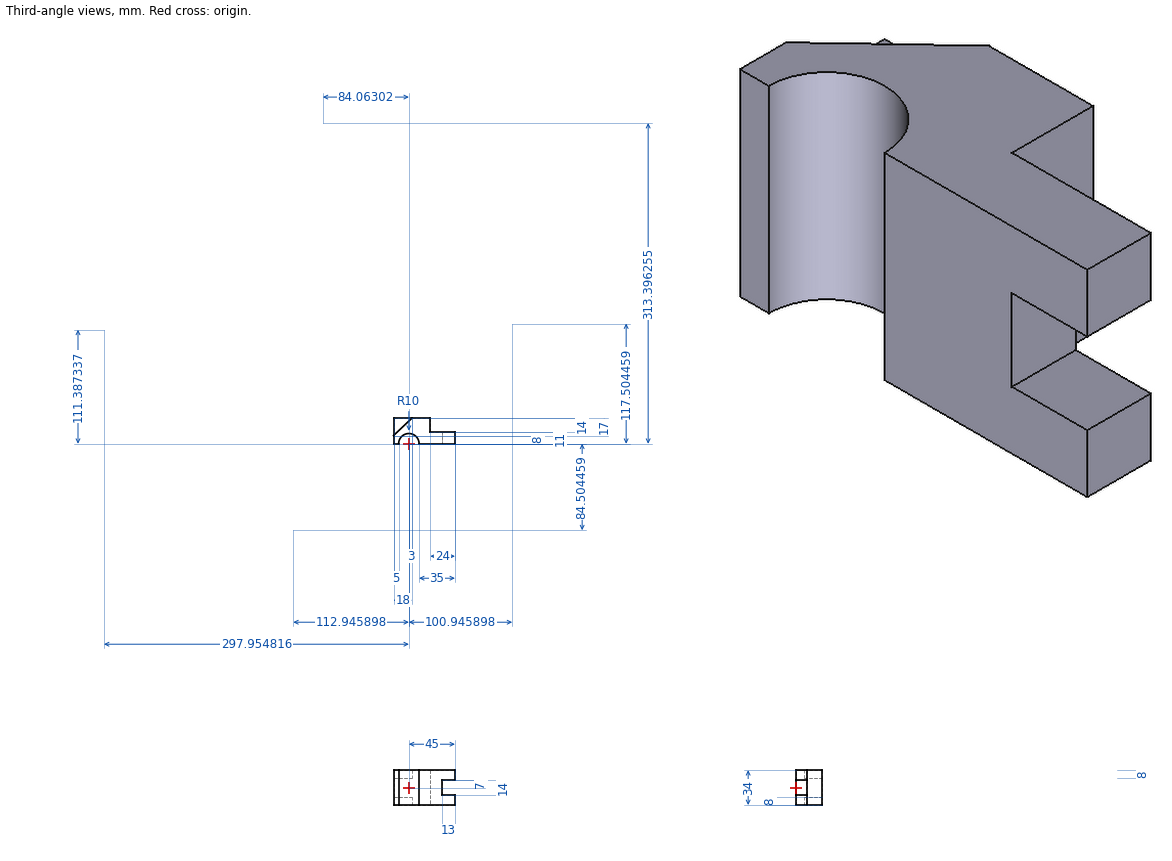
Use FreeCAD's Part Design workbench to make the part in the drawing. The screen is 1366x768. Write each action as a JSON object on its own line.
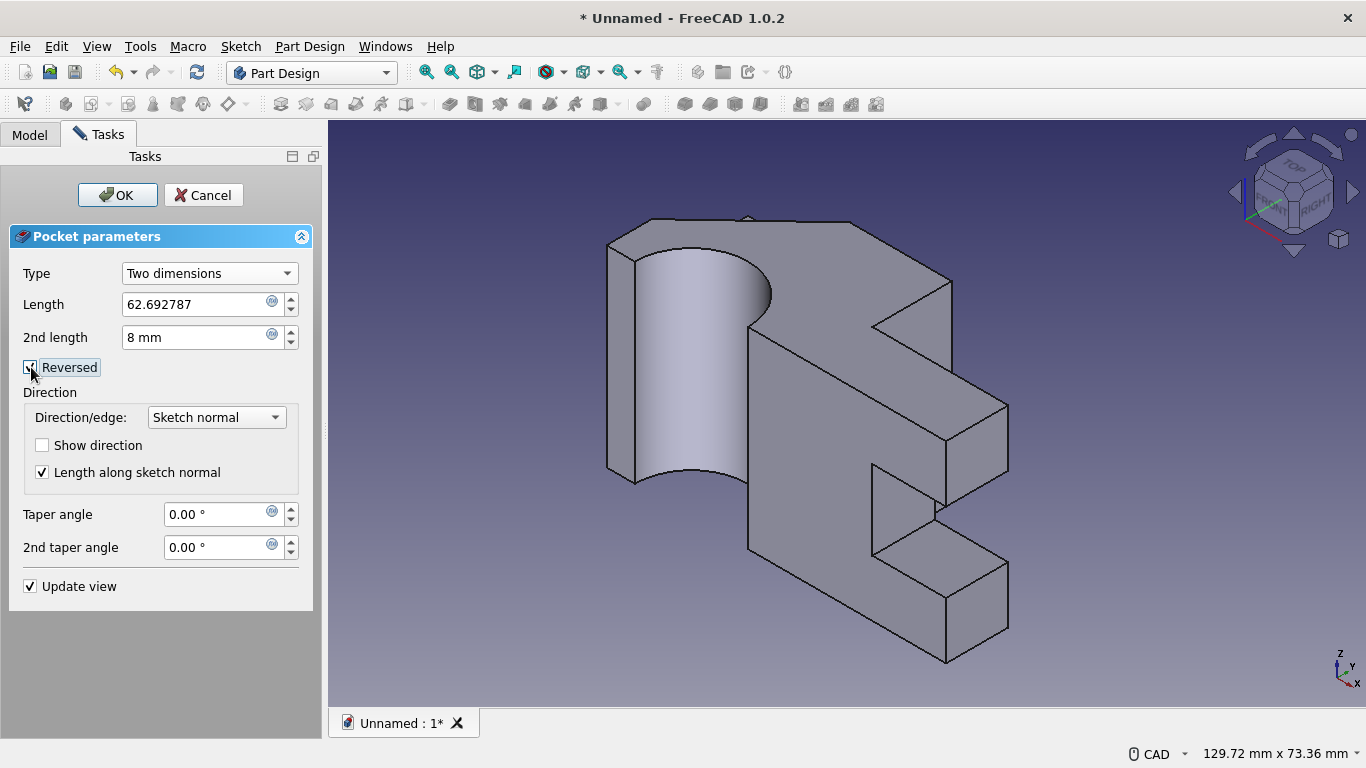
{"action": "left_click", "coordinate": [118, 195]}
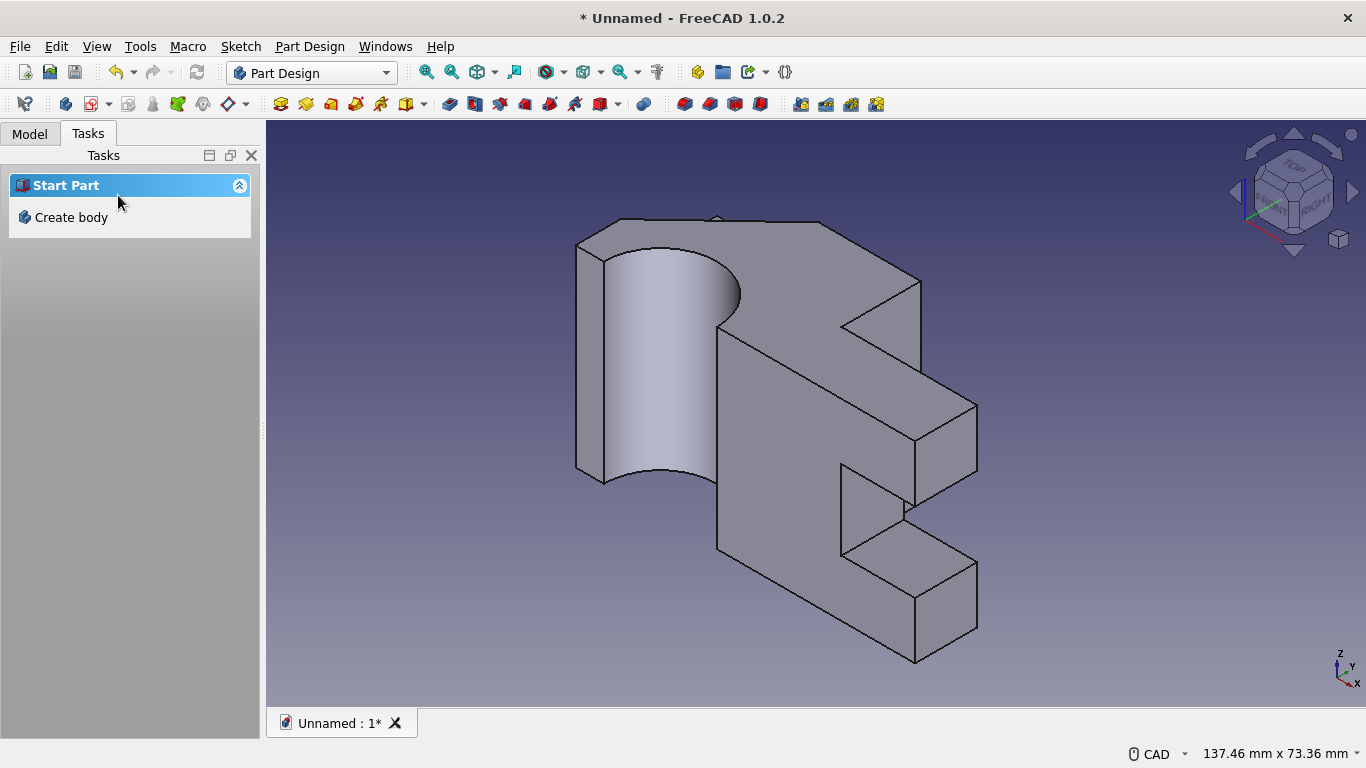
{"action": "key", "text": "5"}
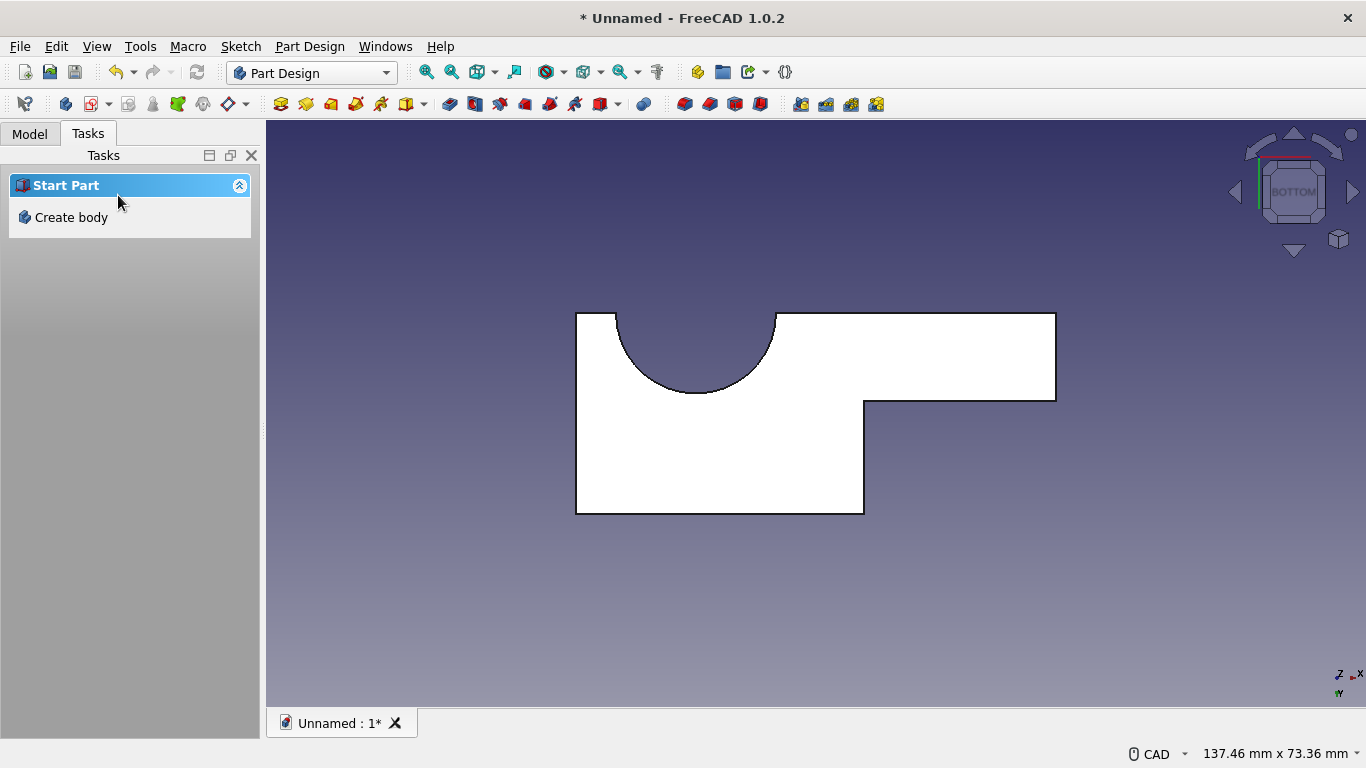
{"action": "left_click", "coordinate": [427, 72]}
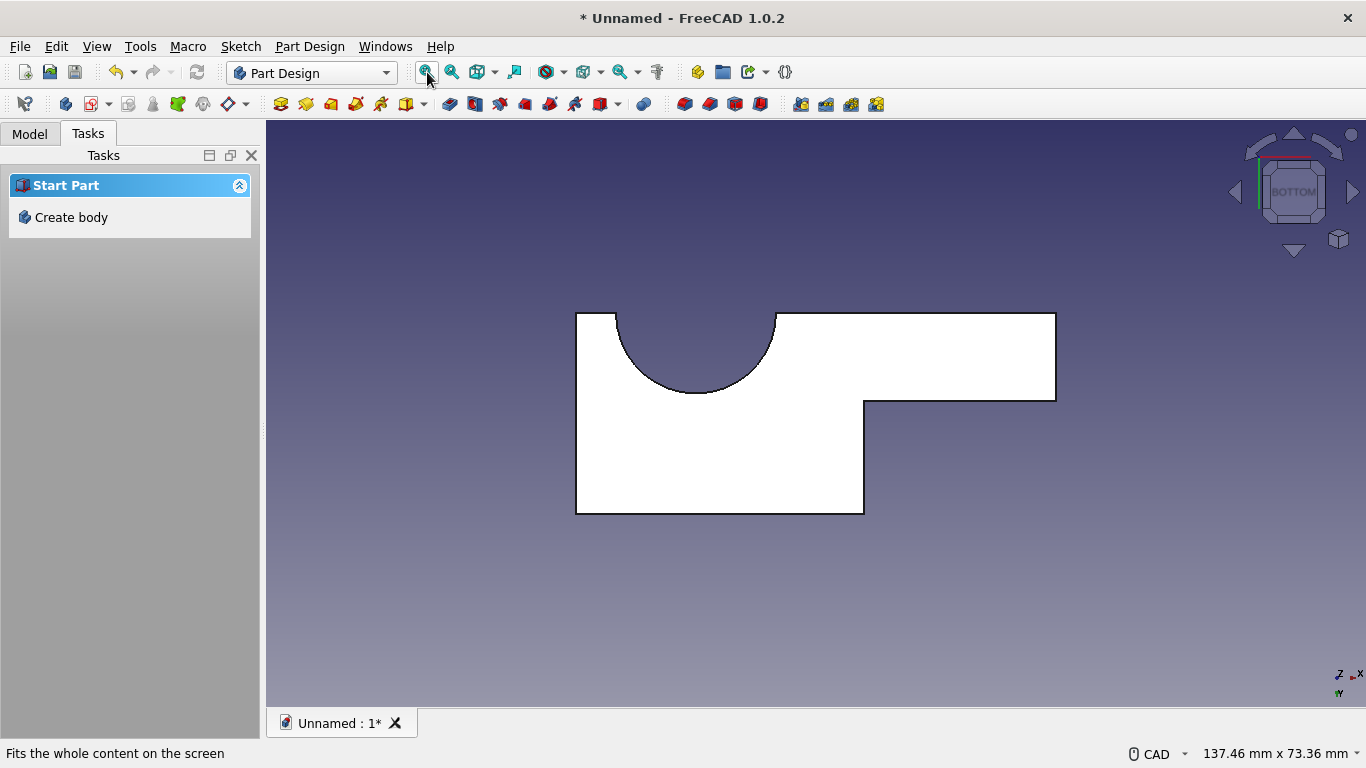
{"action": "left_click", "coordinate": [747, 441]}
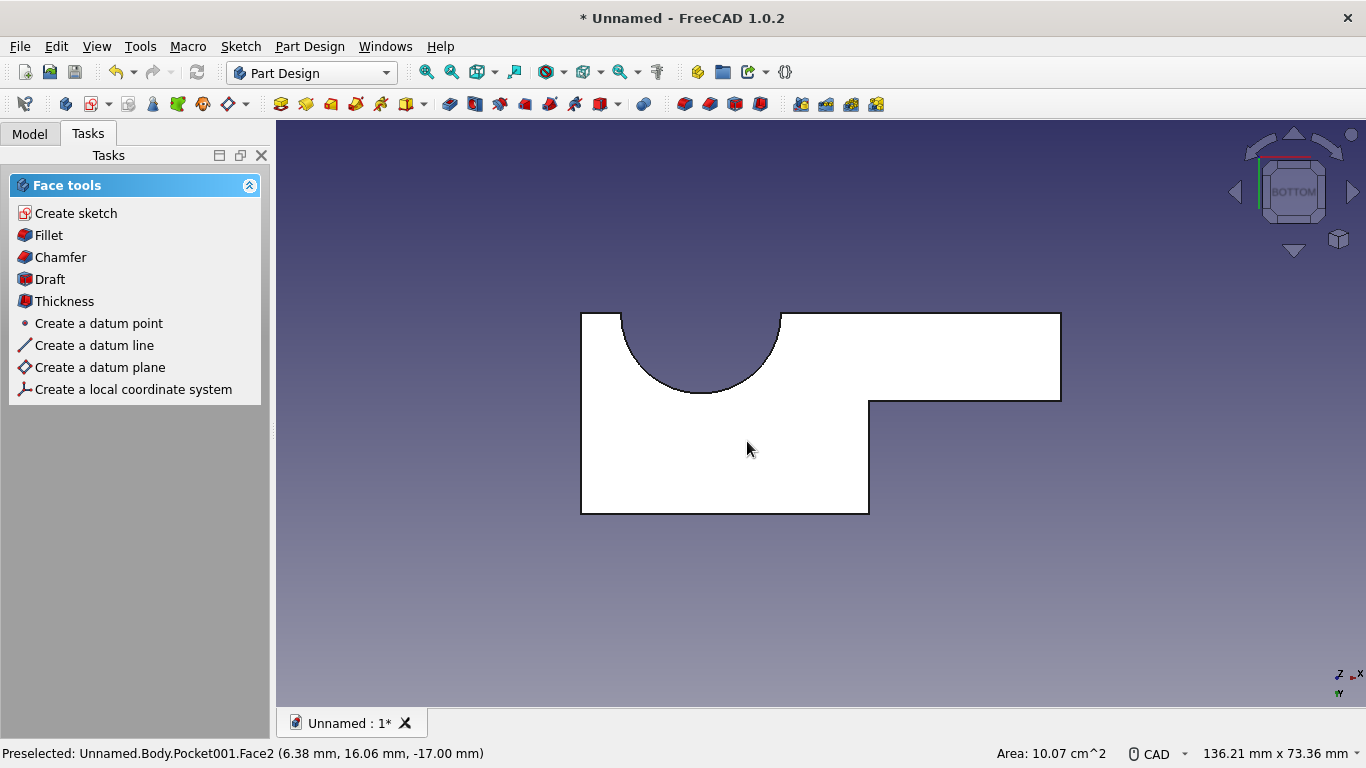
{"action": "left_click", "coordinate": [90, 104]}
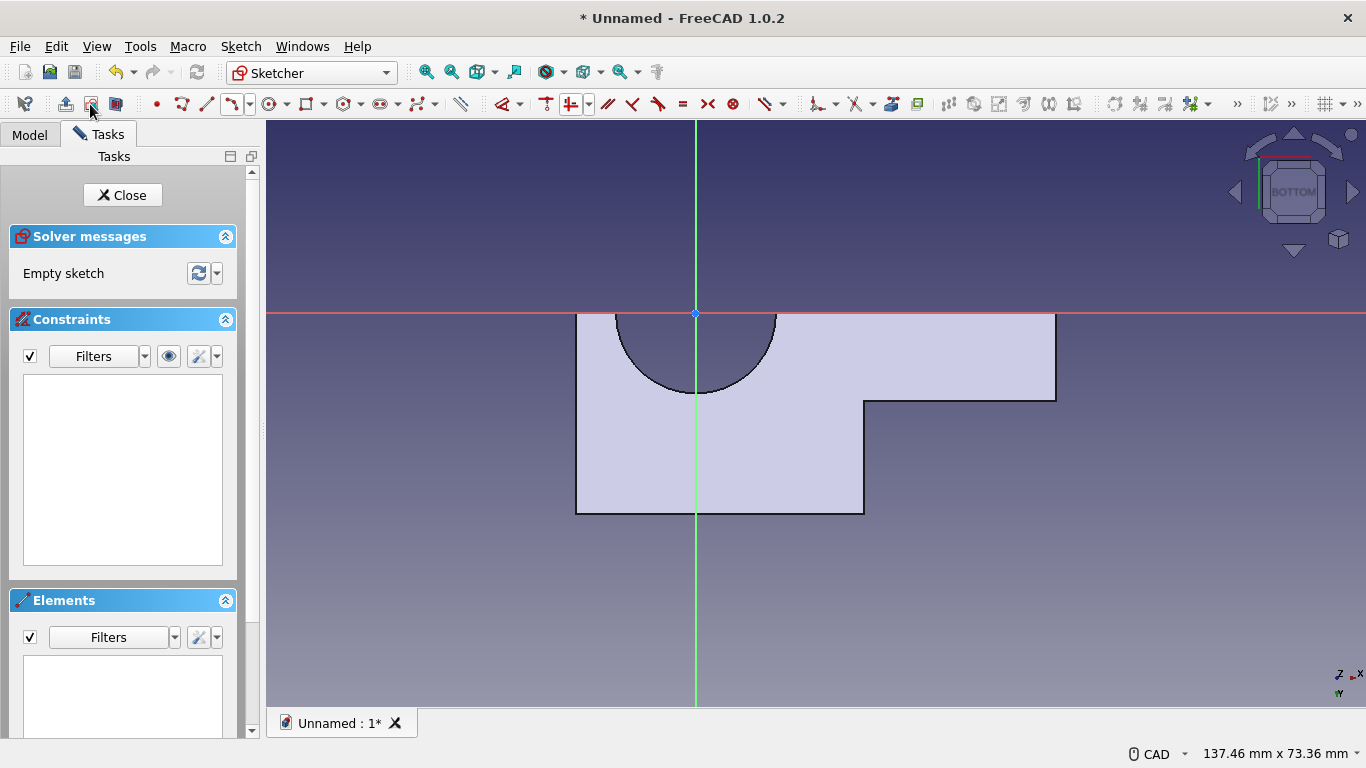
{"action": "scroll", "coordinate": [527, 414], "scroll_direction": "up", "scroll_amount": 3}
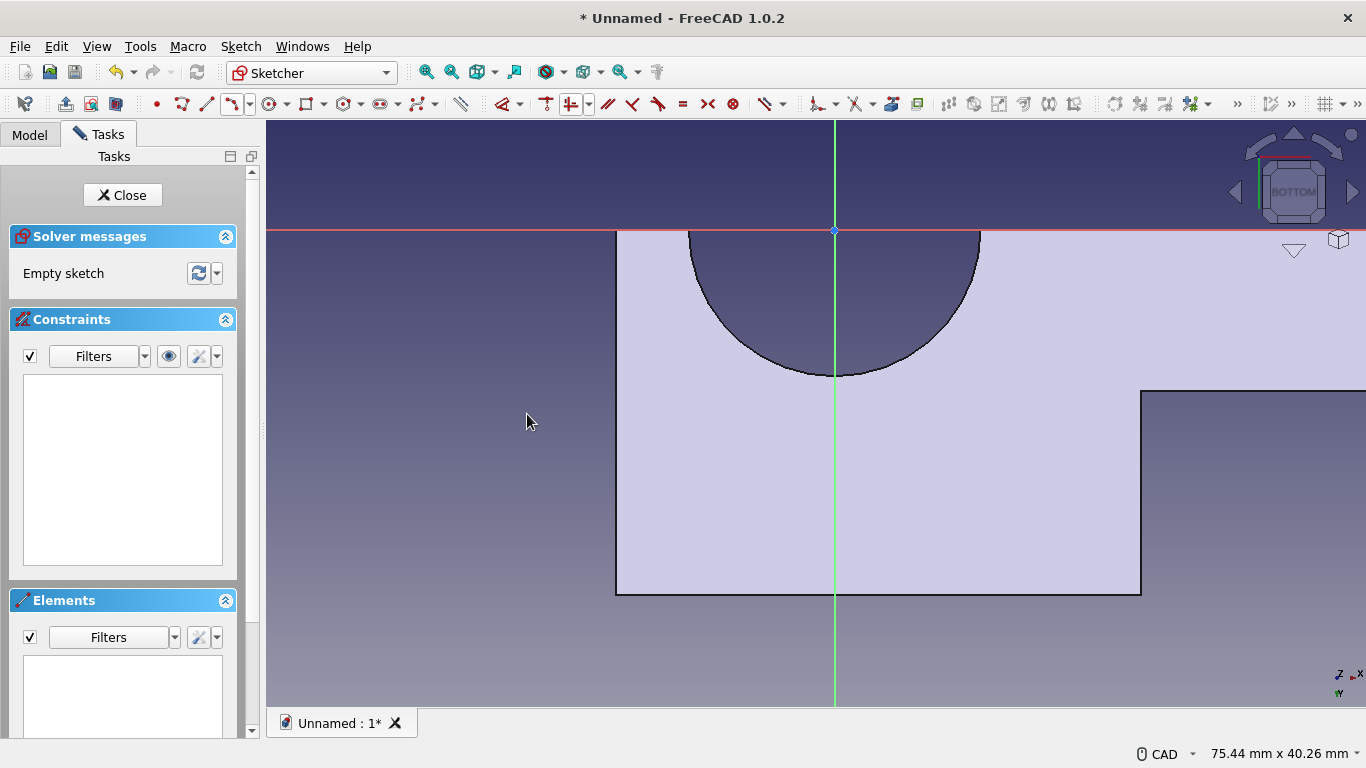
{"action": "left_click", "coordinate": [182, 104]}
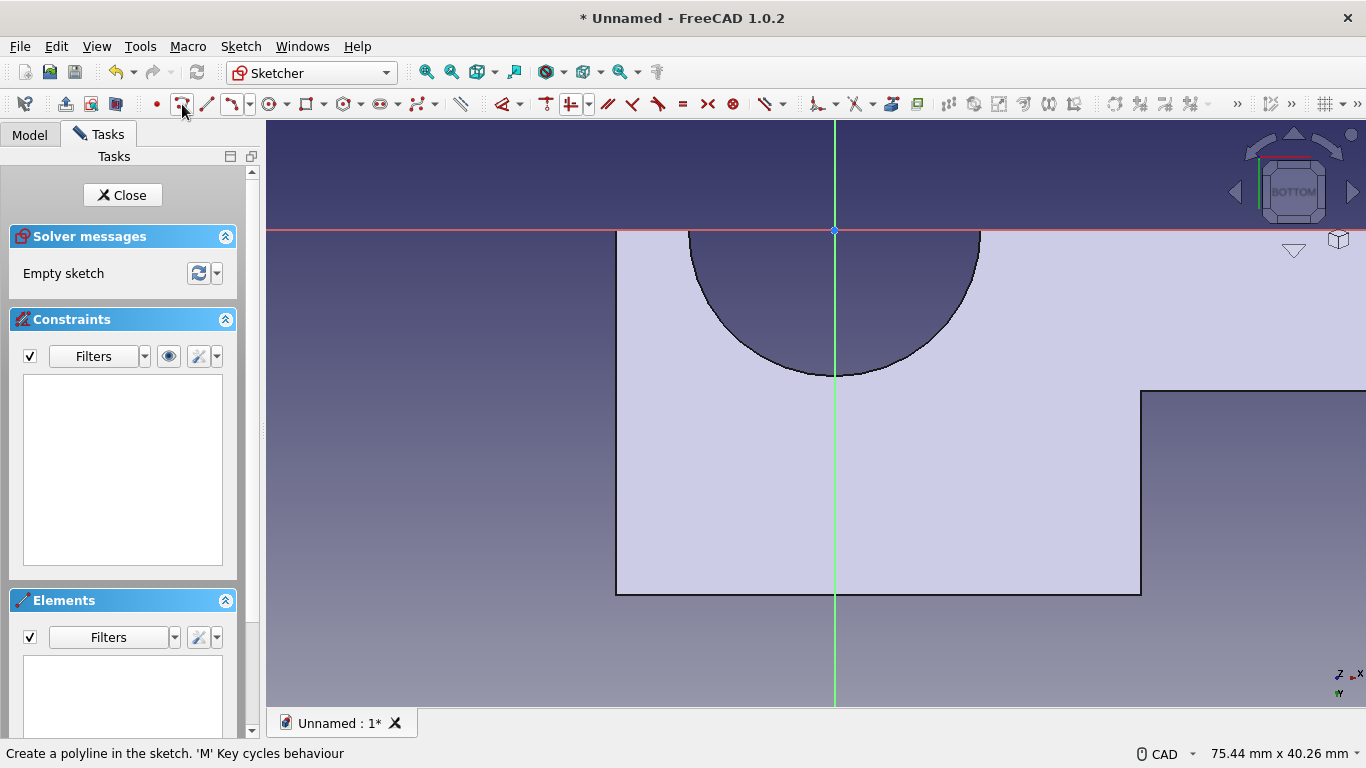
{"action": "left_click", "coordinate": [616, 347]}
{"action": "left_click", "coordinate": [616, 595]}
{"action": "left_click", "coordinate": [878, 595]}
{"action": "left_click", "coordinate": [616, 348]}
{"action": "key", "text": "Escape"}
{"action": "key", "text": "Escape"}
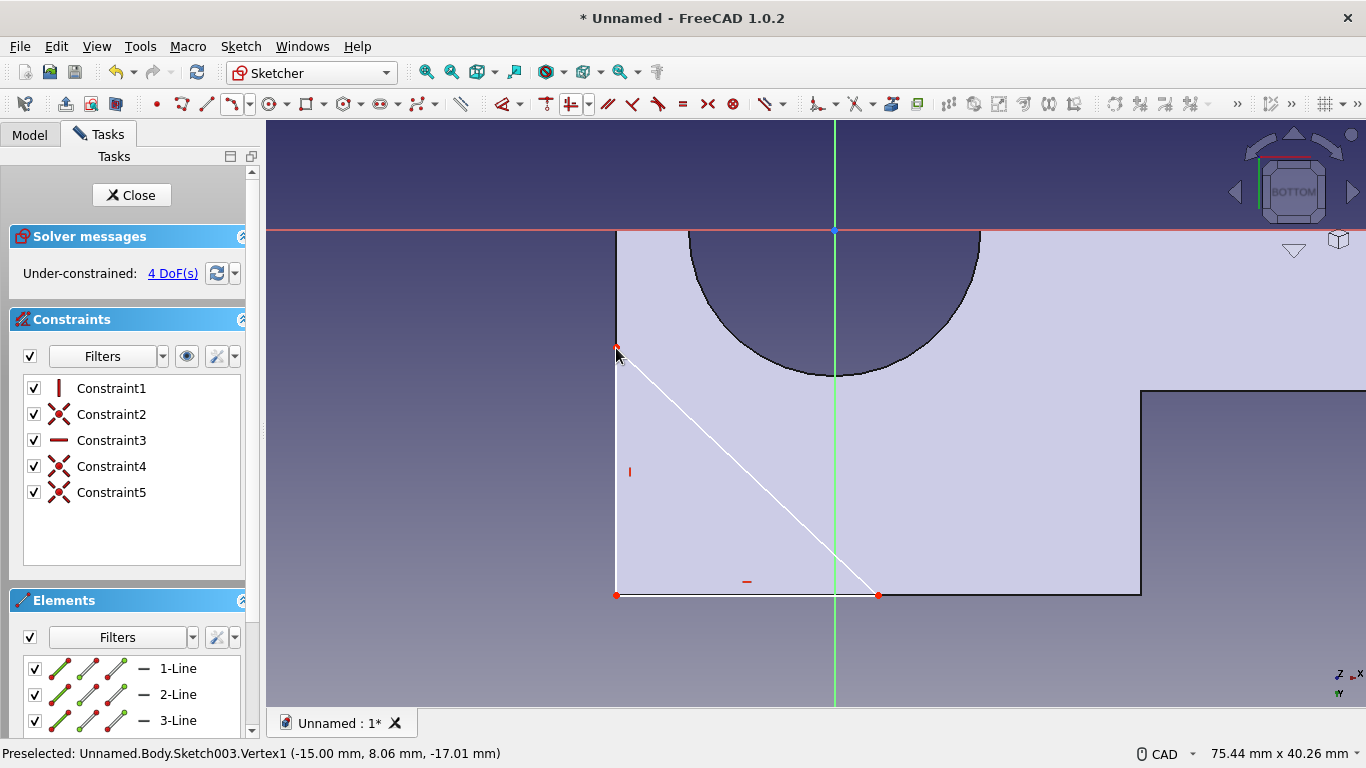
{"action": "left_click", "coordinate": [502, 104]}